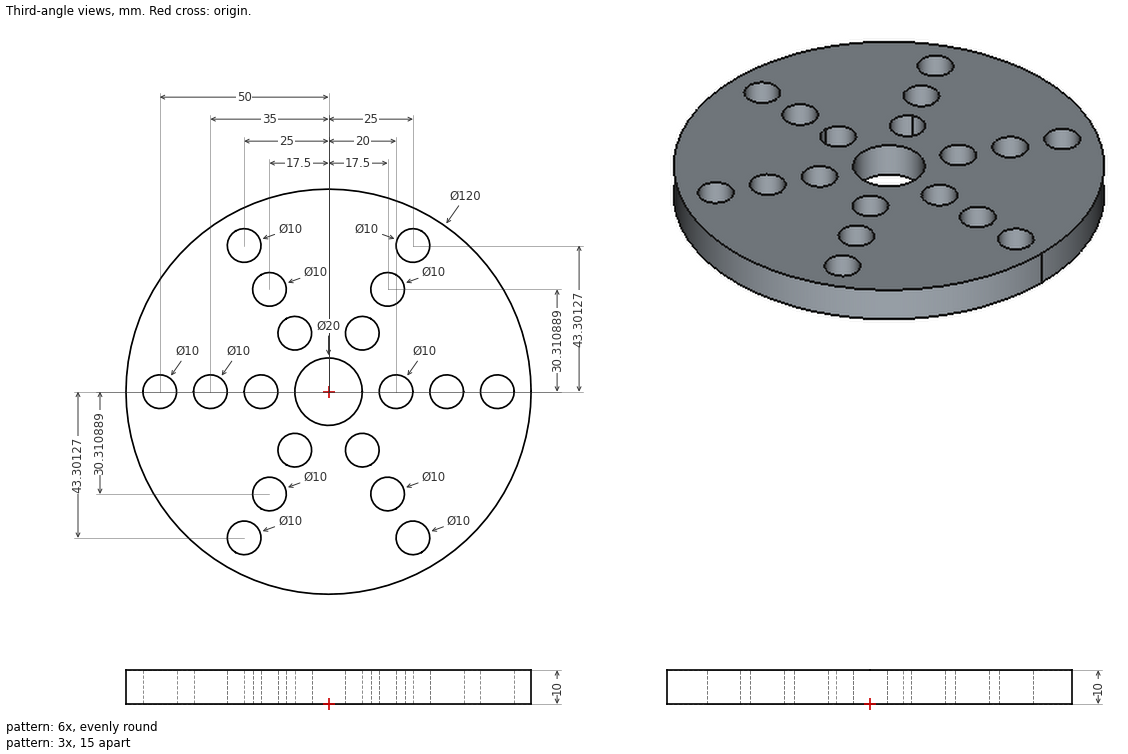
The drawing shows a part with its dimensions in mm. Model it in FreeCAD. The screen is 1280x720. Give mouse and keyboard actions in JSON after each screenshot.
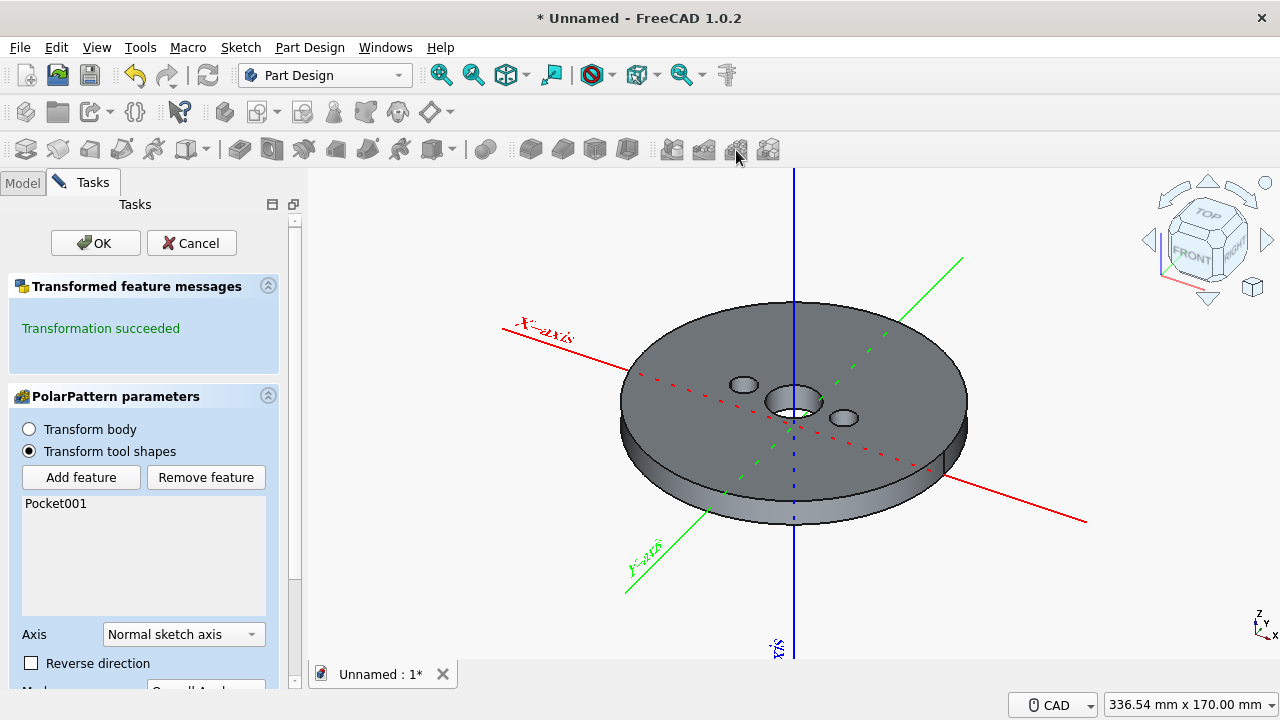
{"action": "left_click", "coordinate": [184, 634]}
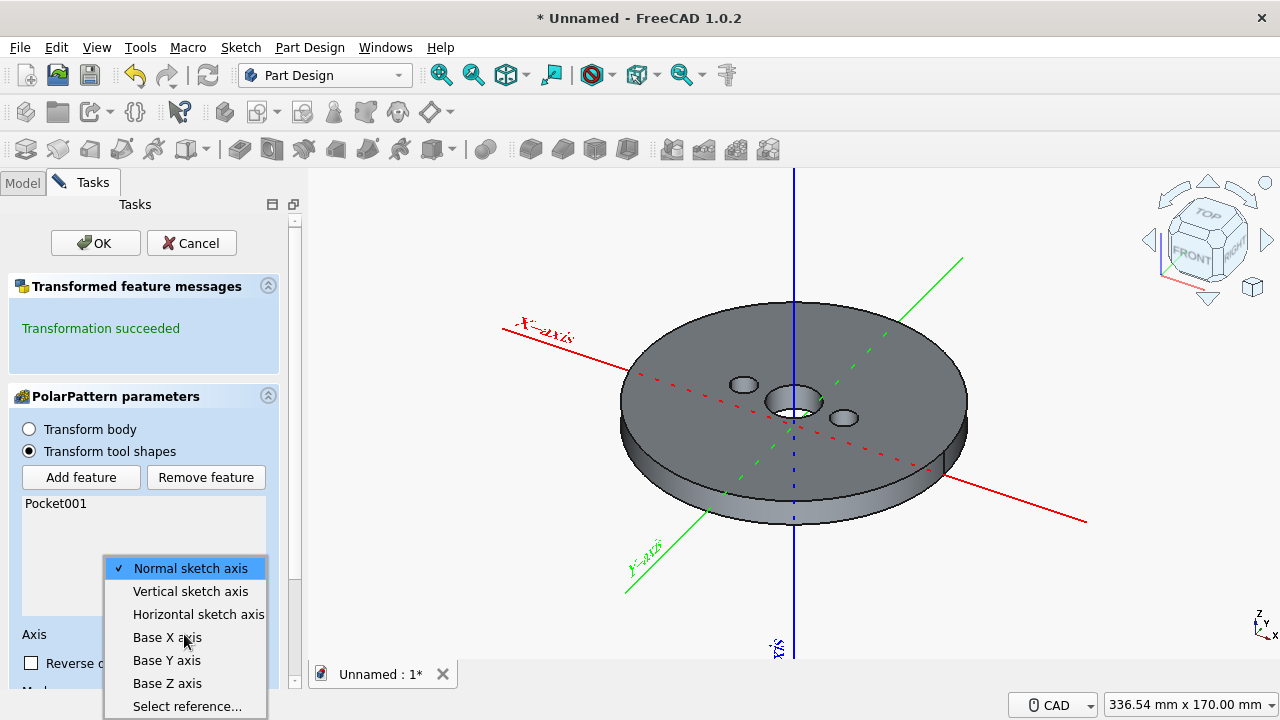
{"action": "left_click", "coordinate": [184, 684]}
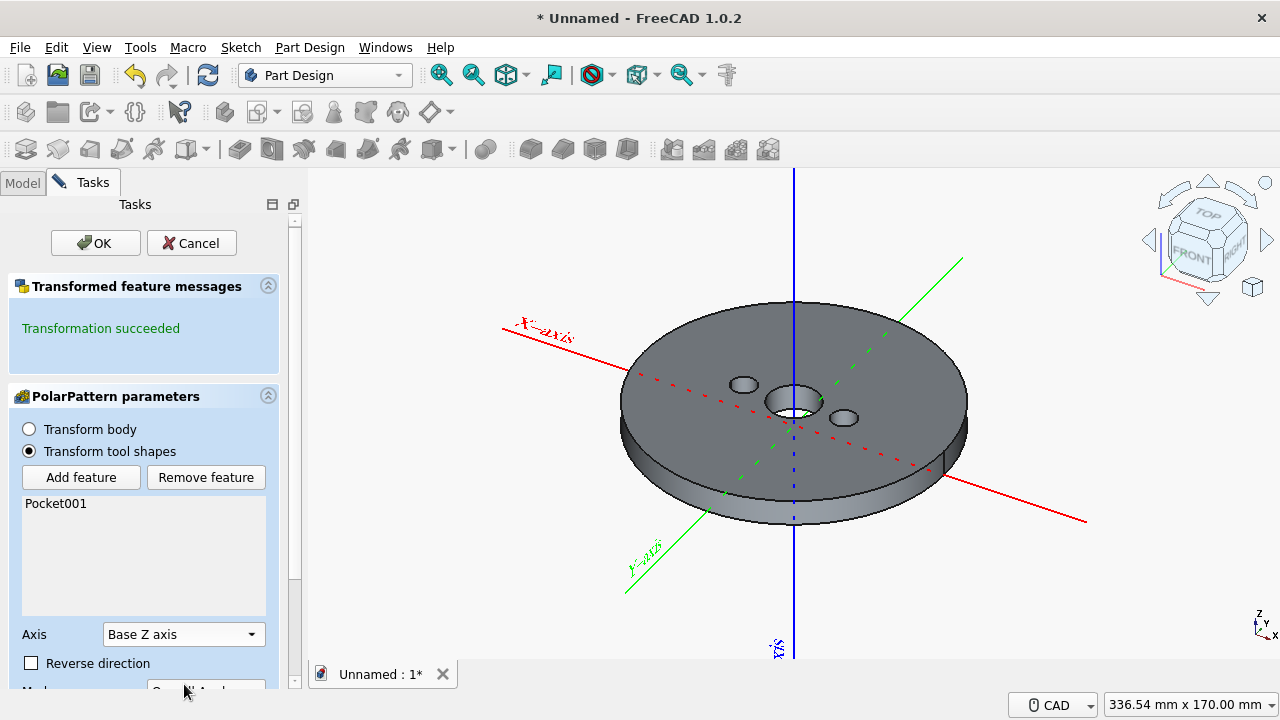
{"action": "scroll", "coordinate": [295, 451], "scroll_direction": "down", "scroll_amount": 3}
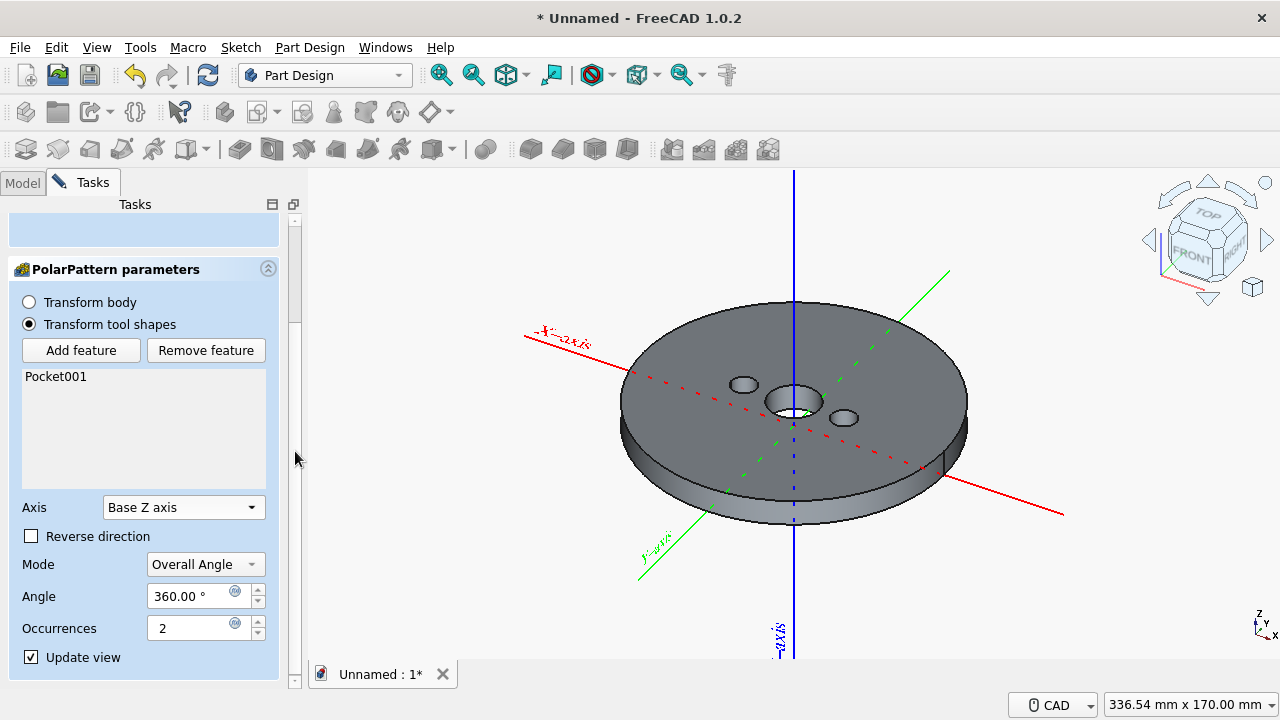
{"action": "triple_click", "coordinate": [198, 628]}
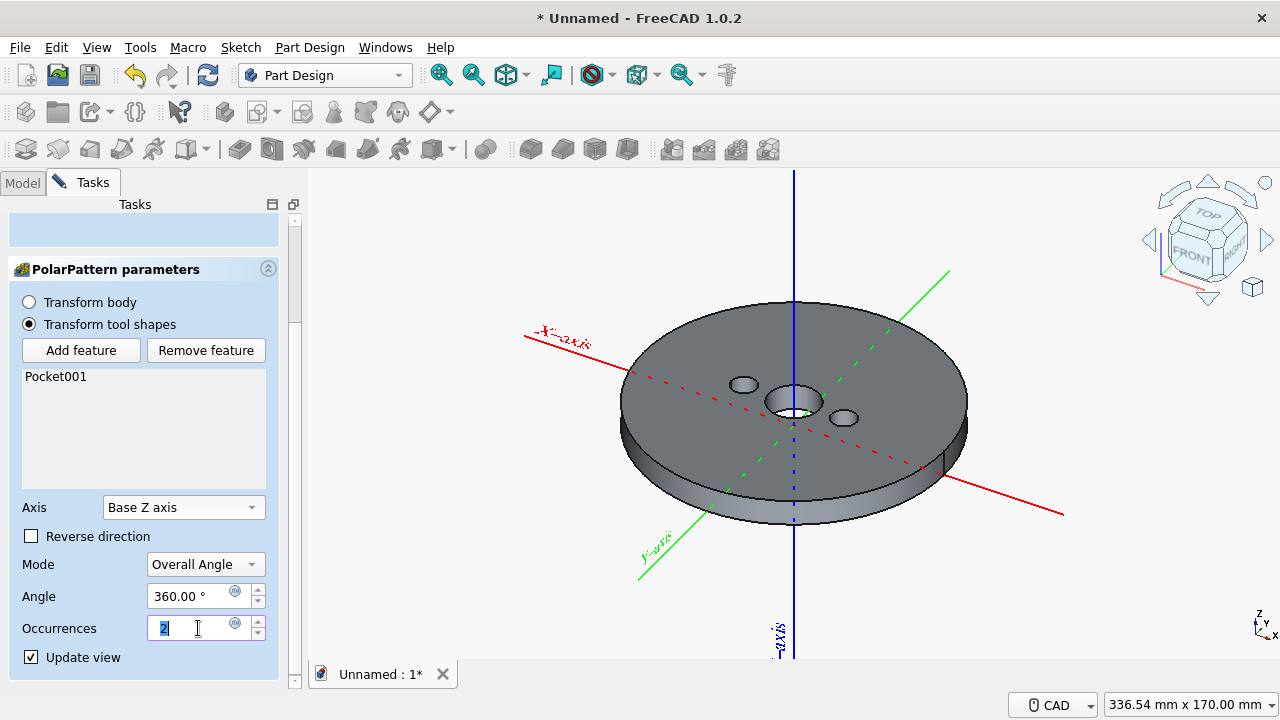
{"action": "type", "text": "6"}
{"action": "key", "text": "Tab"}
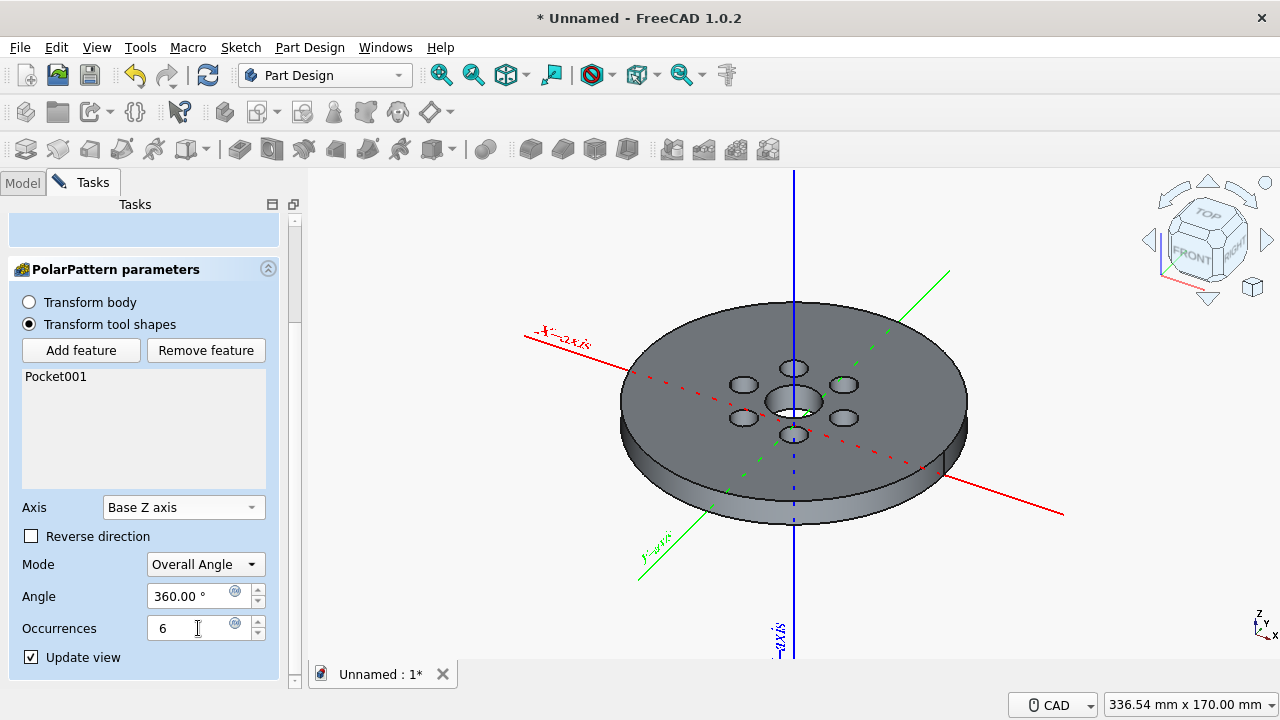
{"action": "scroll", "coordinate": [295, 451], "scroll_direction": "up", "scroll_amount": 3}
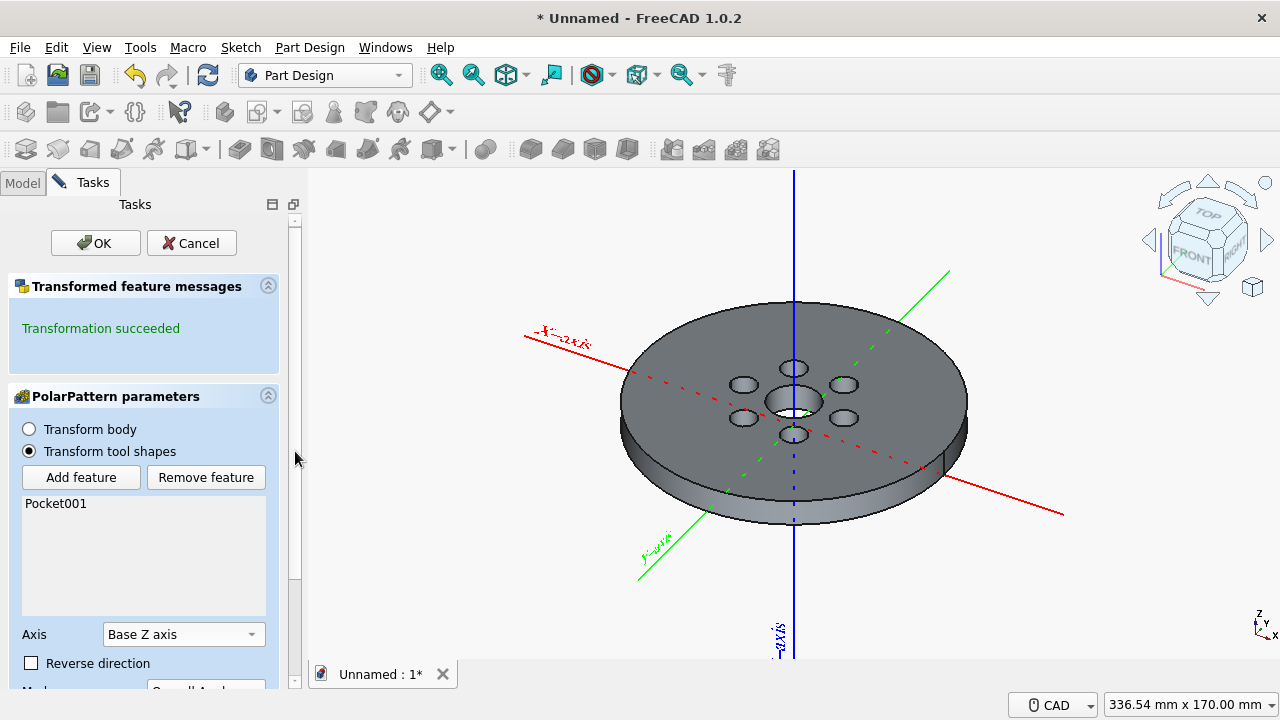
{"action": "left_click", "coordinate": [96, 243]}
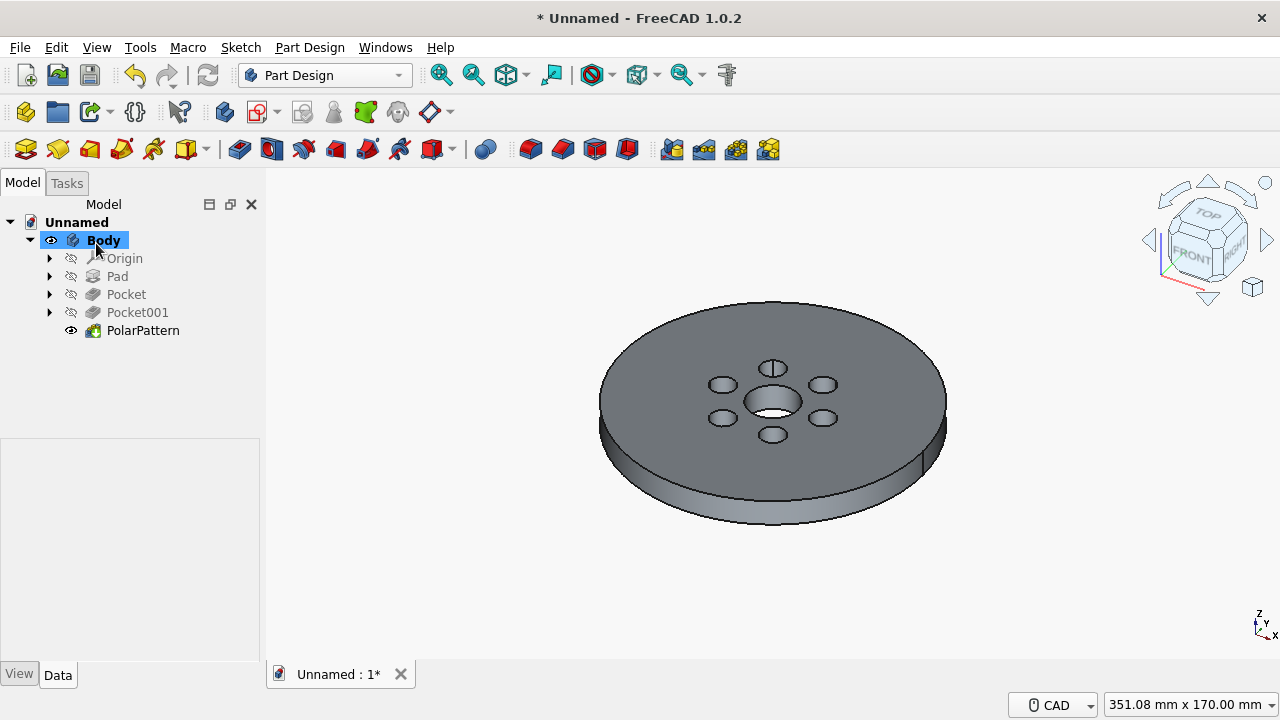
{"action": "left_click", "coordinate": [116, 312]}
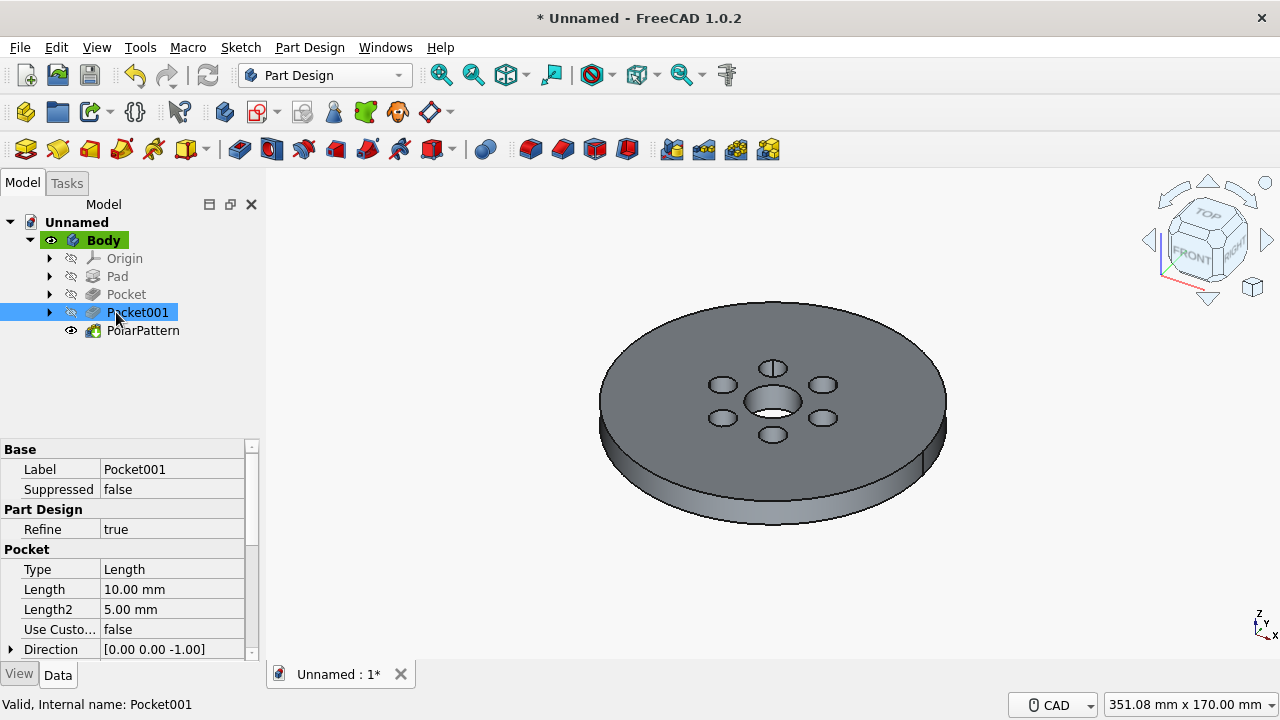
{"action": "left_click", "coordinate": [704, 150]}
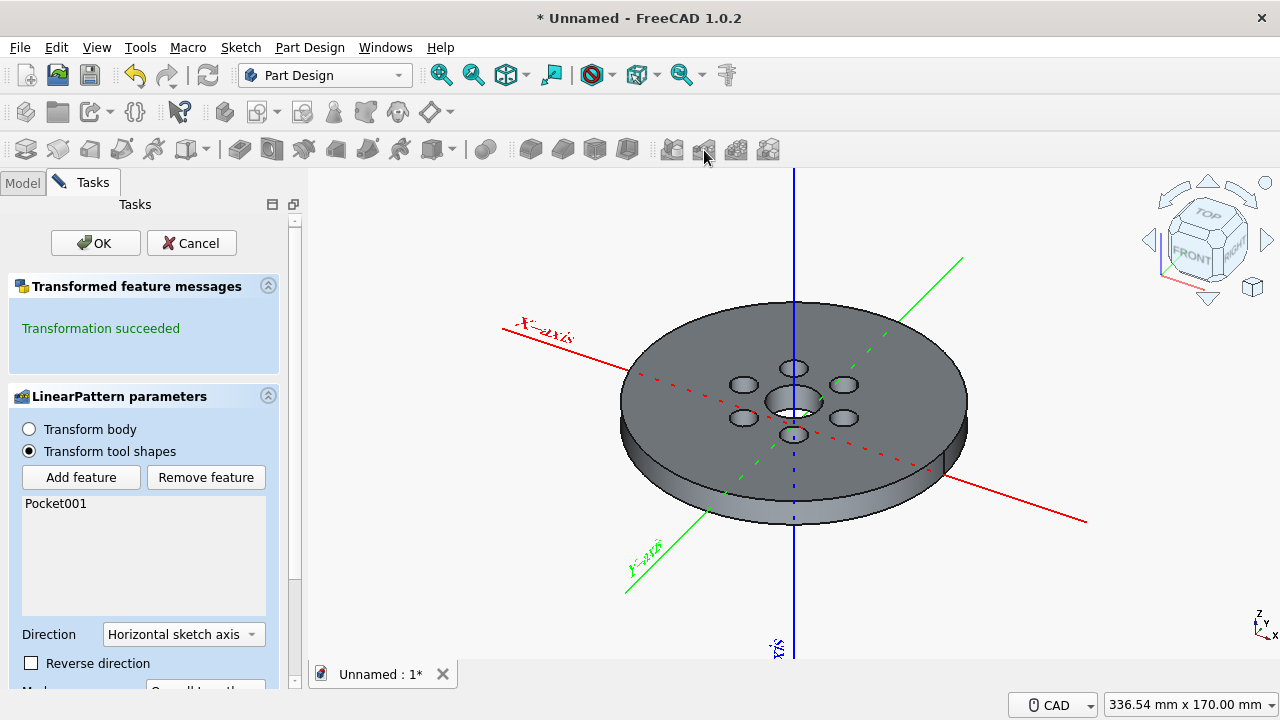
{"action": "left_click", "coordinate": [184, 634]}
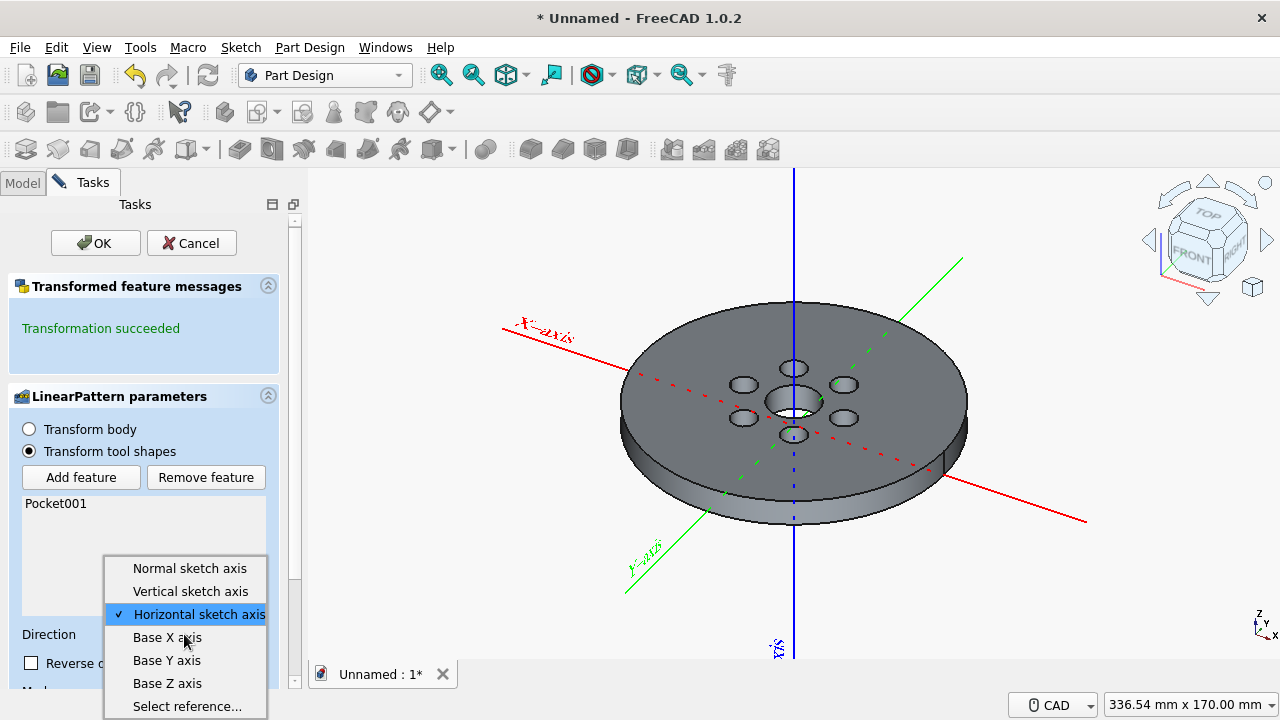
{"action": "left_click", "coordinate": [184, 638]}